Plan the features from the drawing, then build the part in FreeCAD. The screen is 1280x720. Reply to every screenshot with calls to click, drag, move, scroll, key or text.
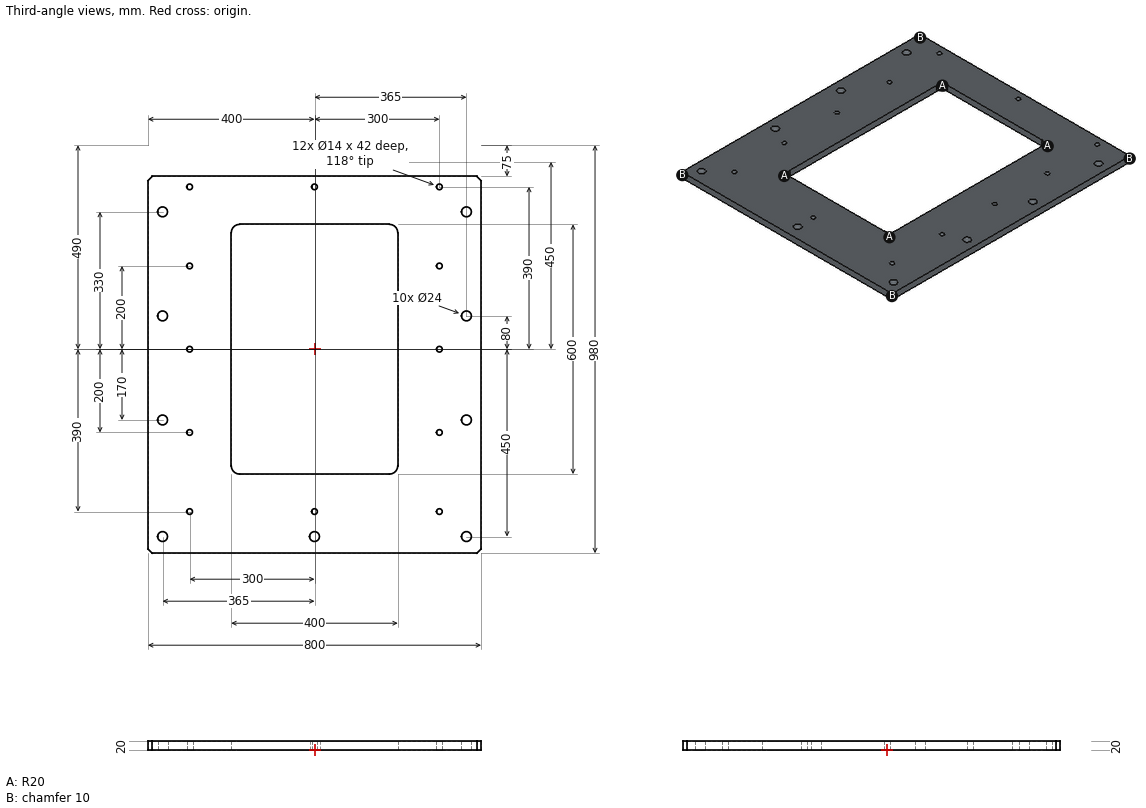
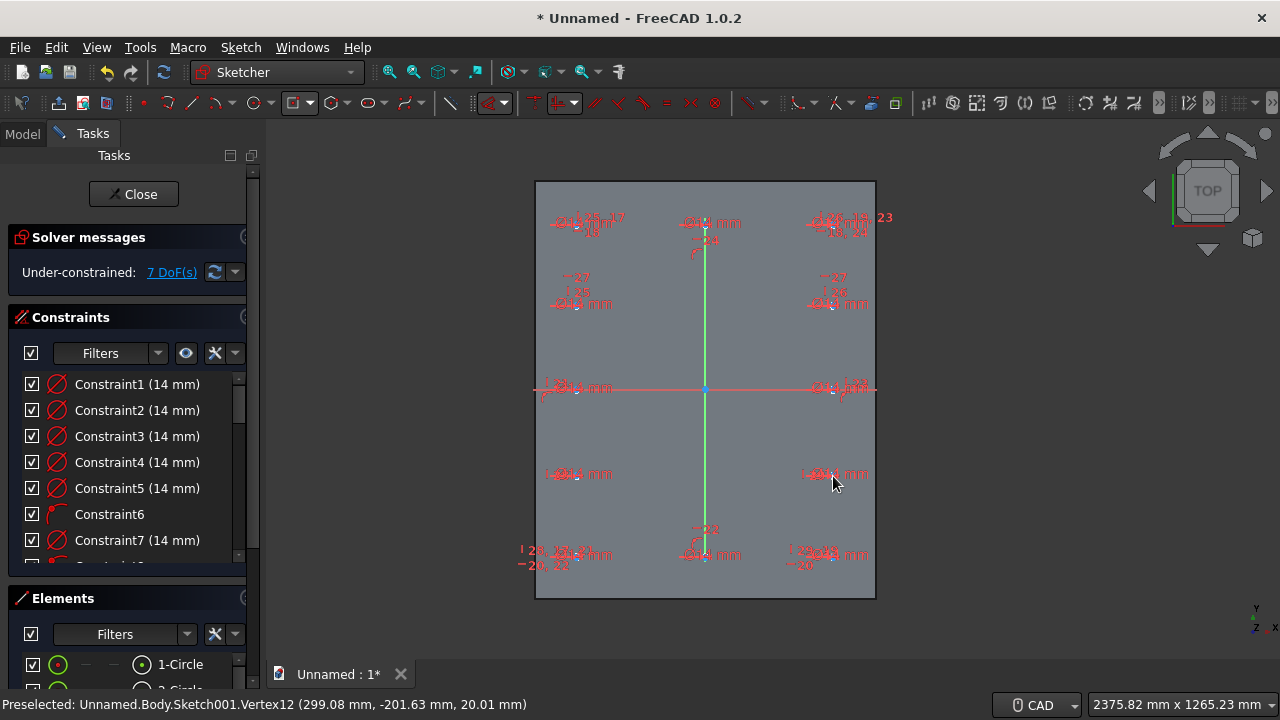
click(577, 476)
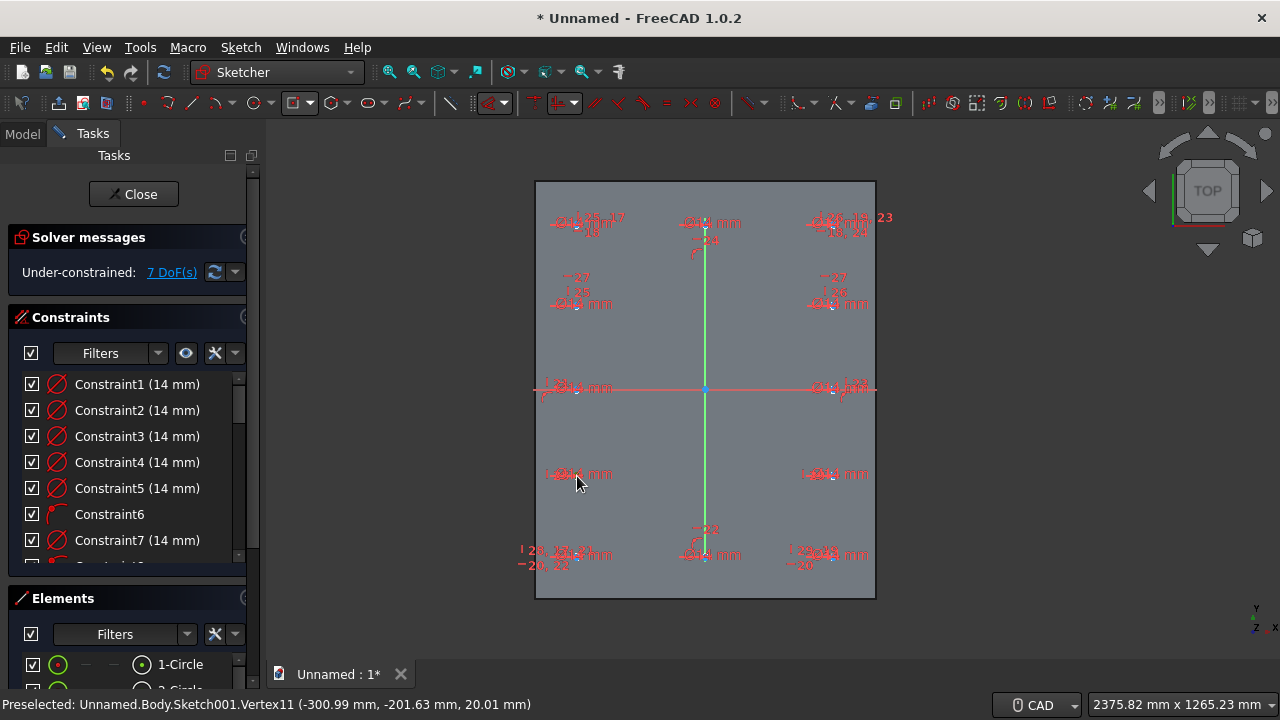
click(833, 476)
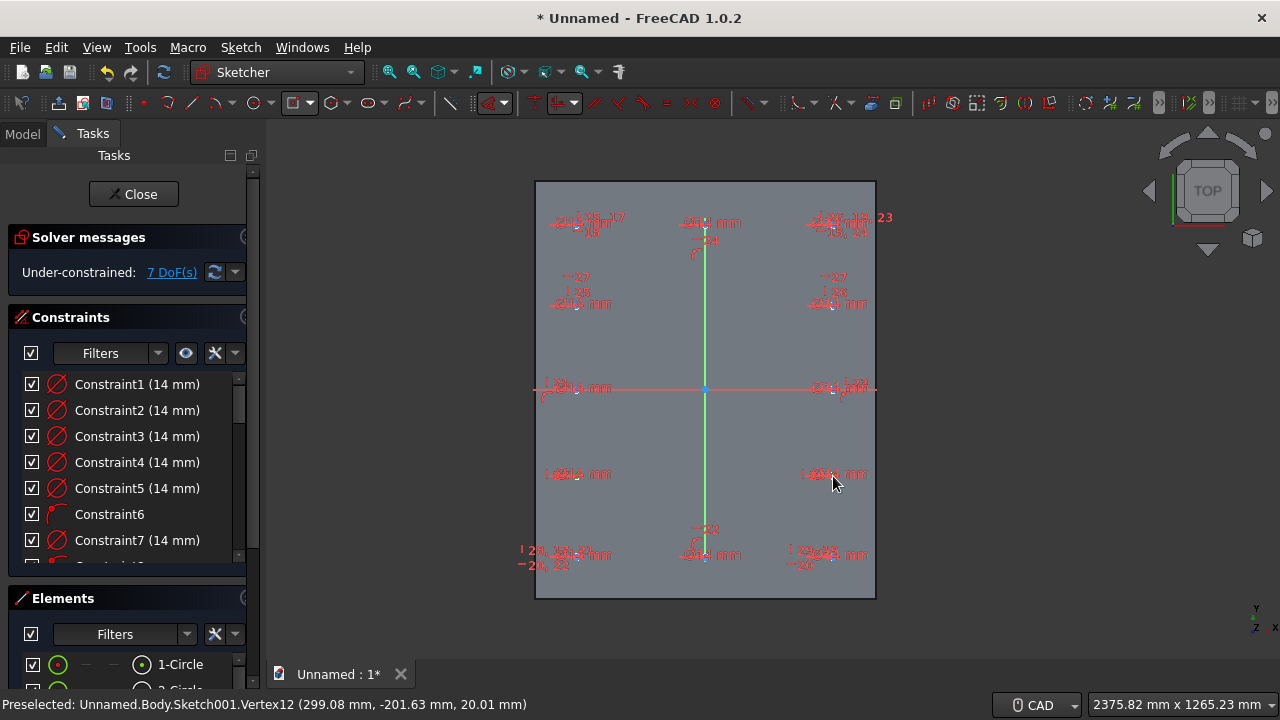
key(h)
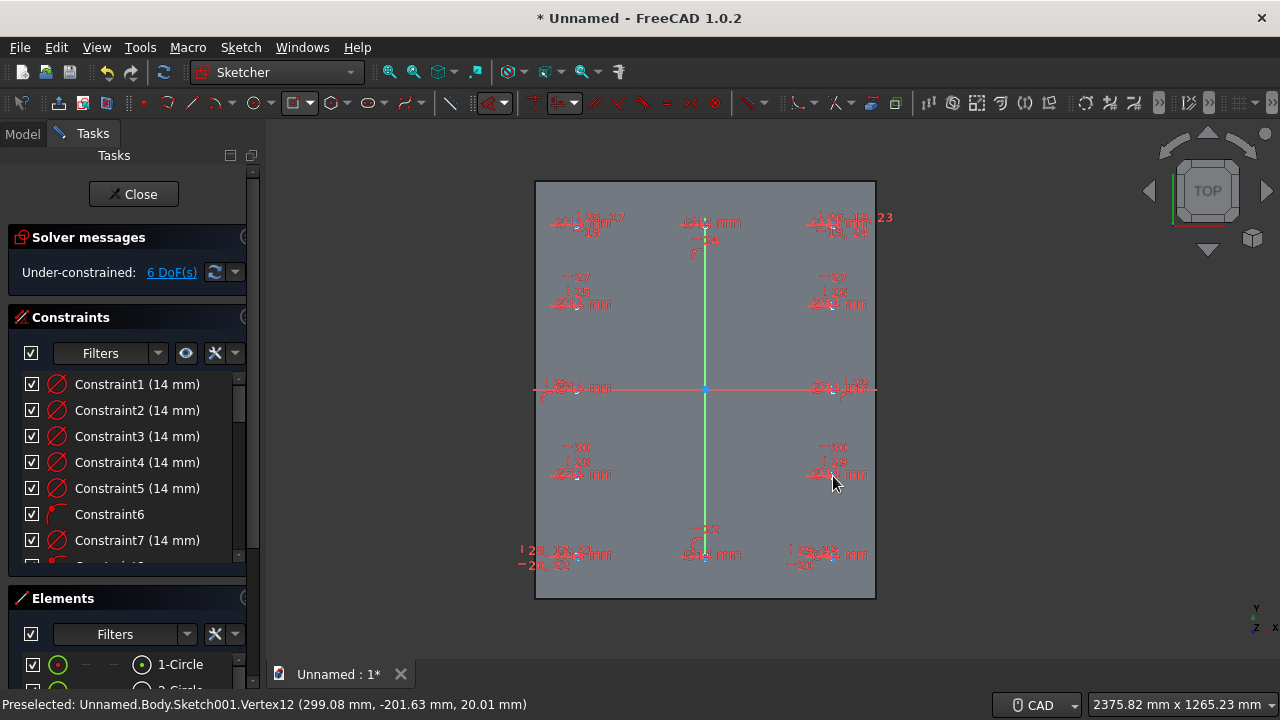
click(488, 104)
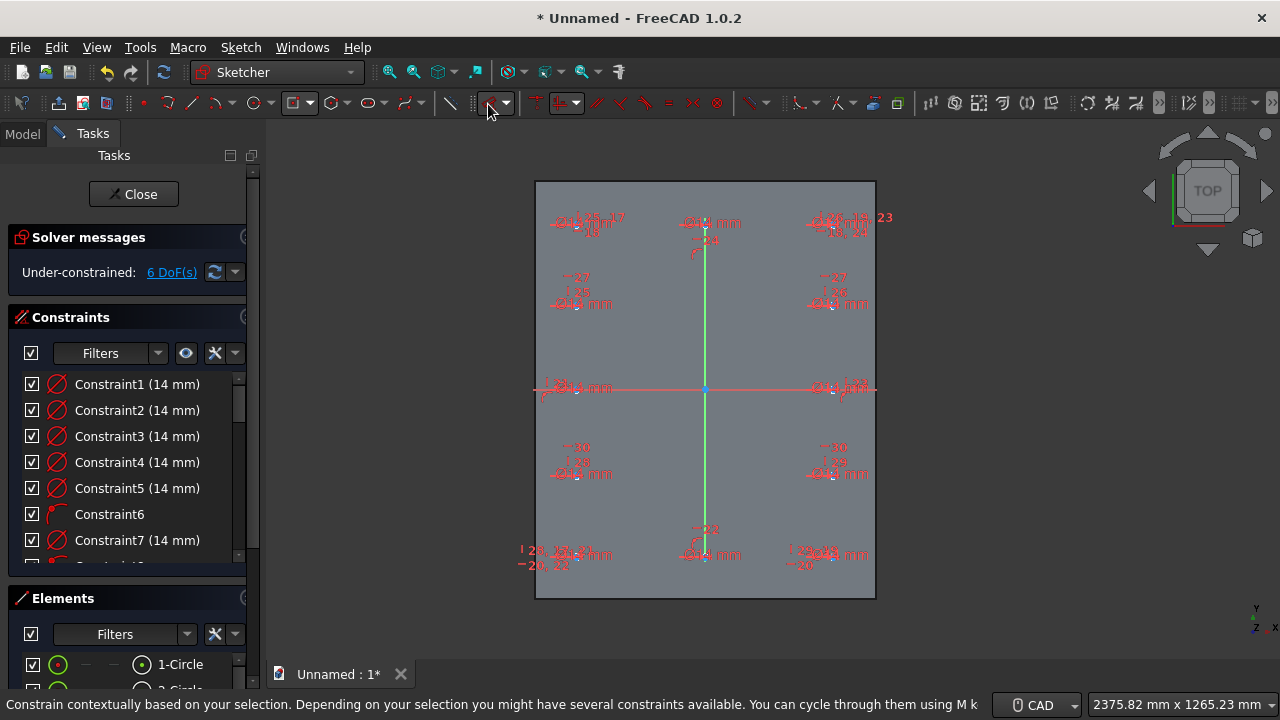
click(833, 225)
click(769, 191)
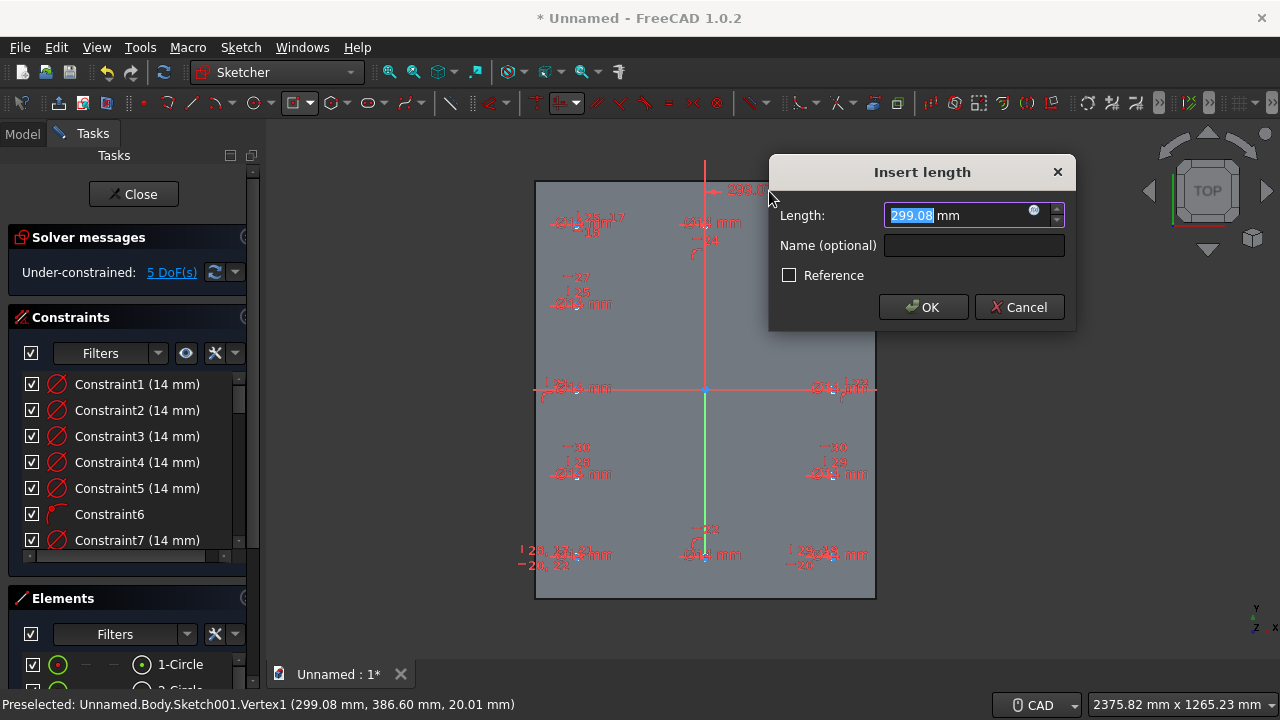
text(300)
key(Return)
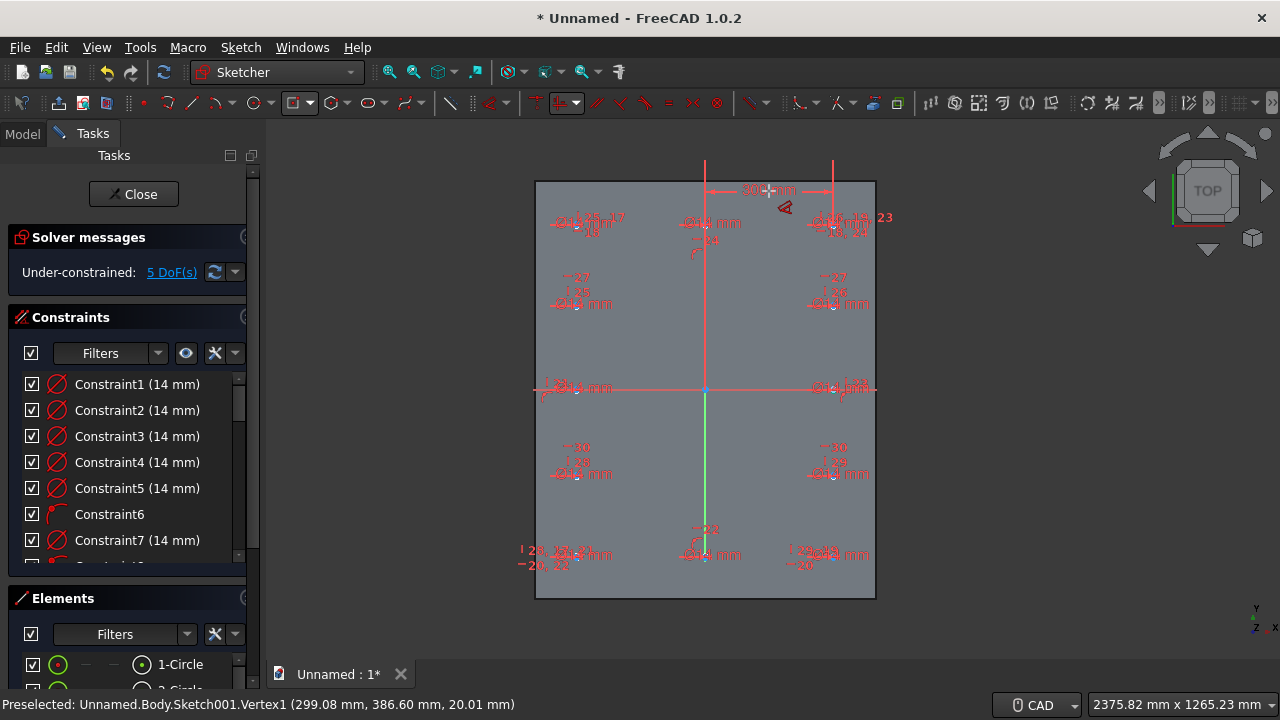
click(833, 225)
click(867, 307)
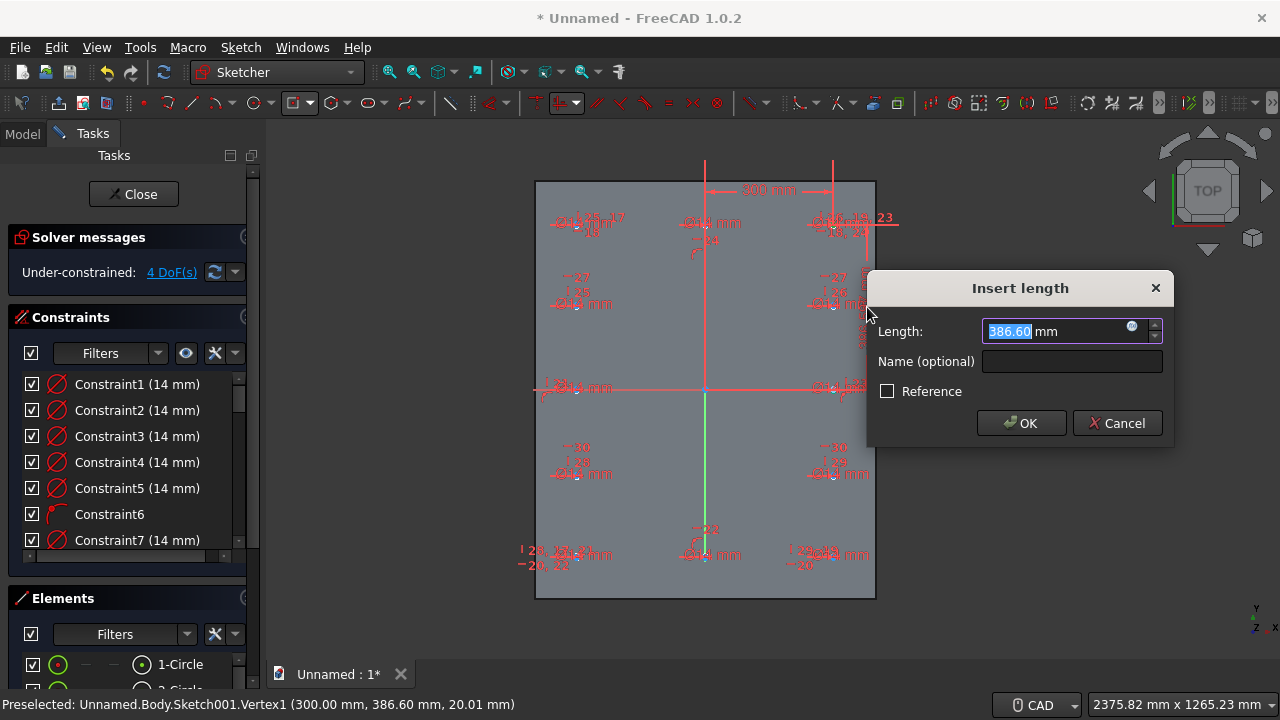
text(390)
key(Return)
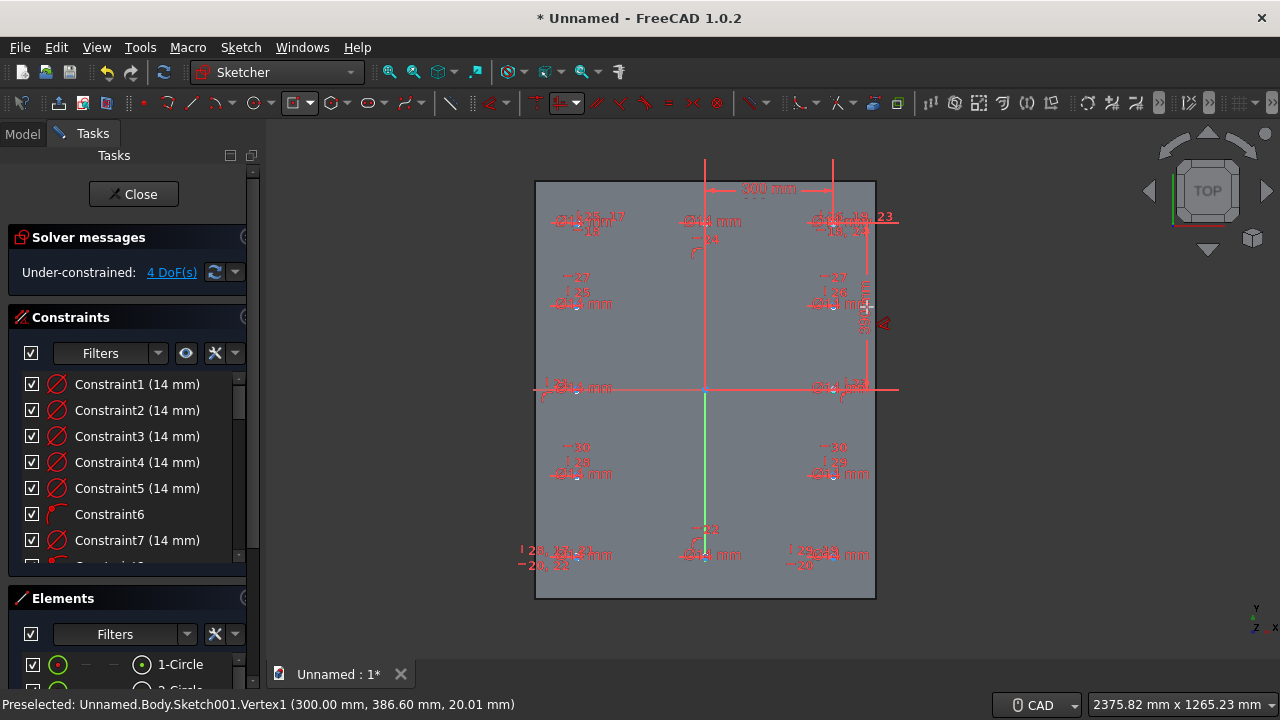
click(577, 557)
click(641, 591)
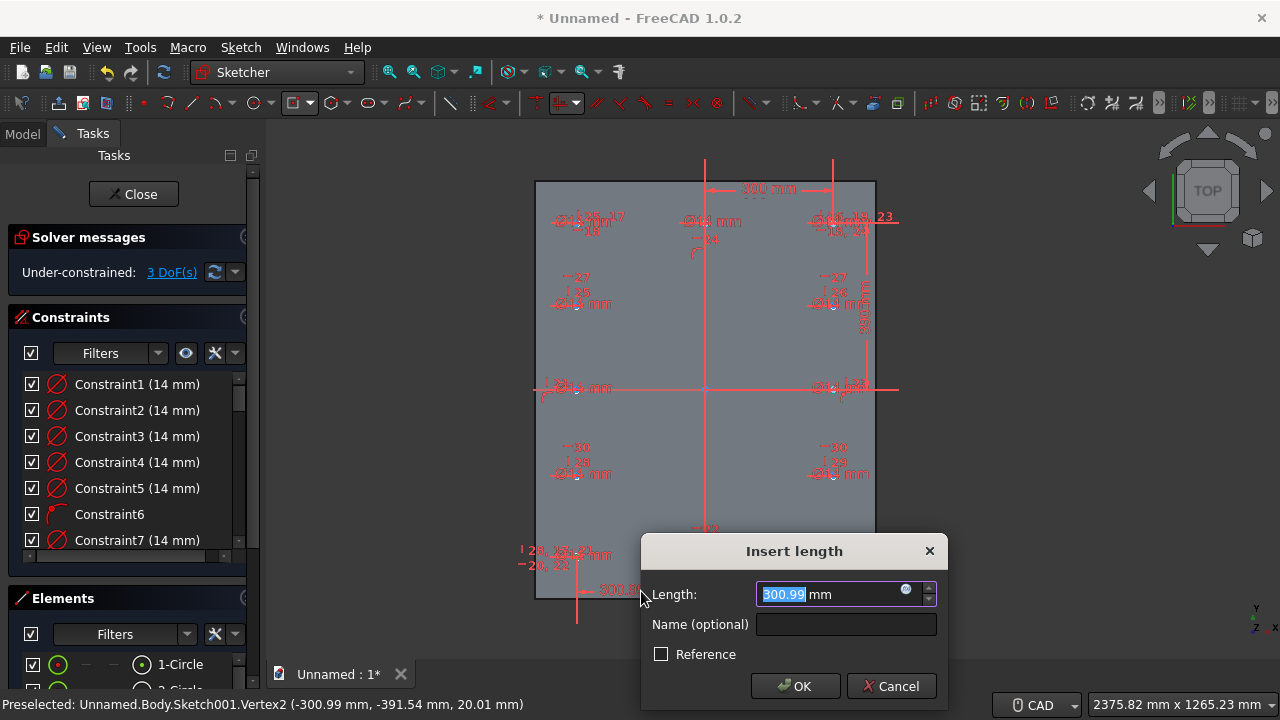
text(300)
key(Return)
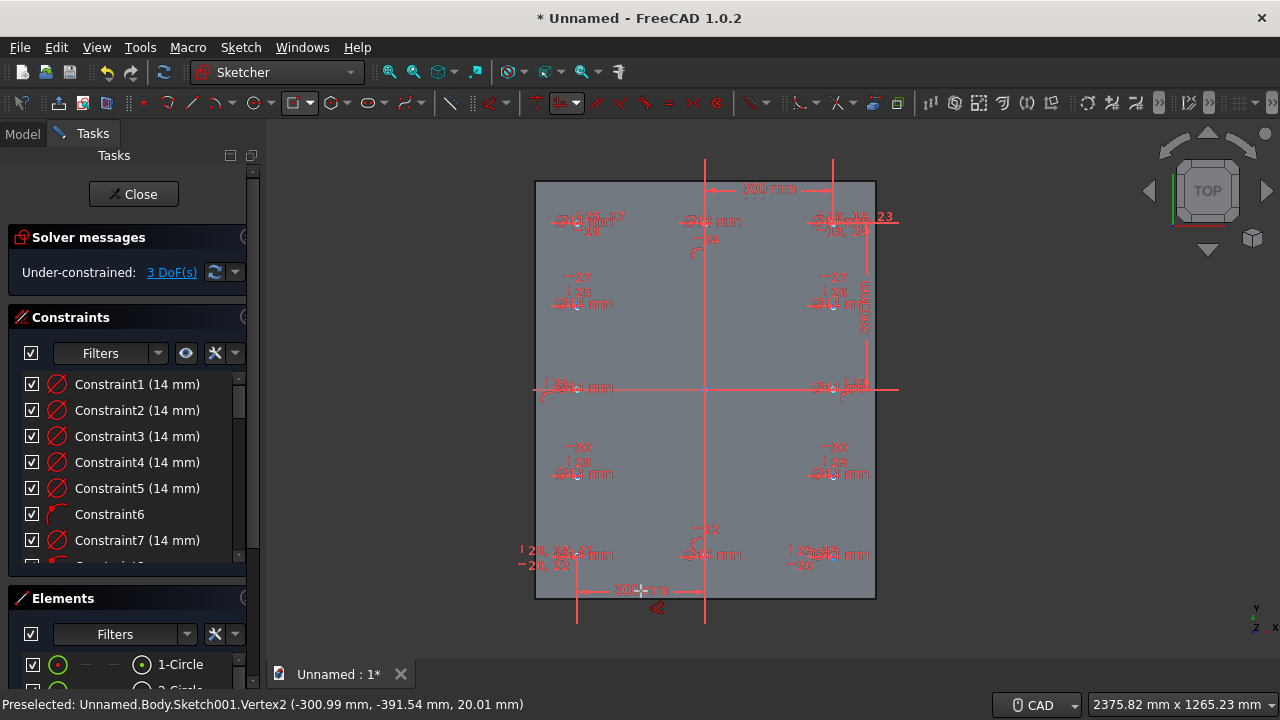
click(577, 557)
click(543, 473)